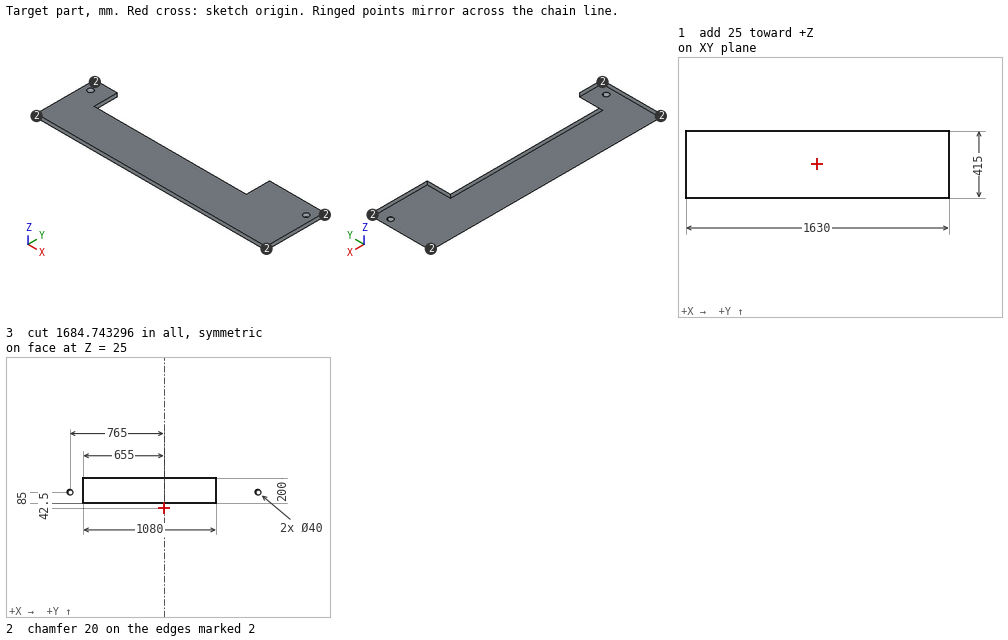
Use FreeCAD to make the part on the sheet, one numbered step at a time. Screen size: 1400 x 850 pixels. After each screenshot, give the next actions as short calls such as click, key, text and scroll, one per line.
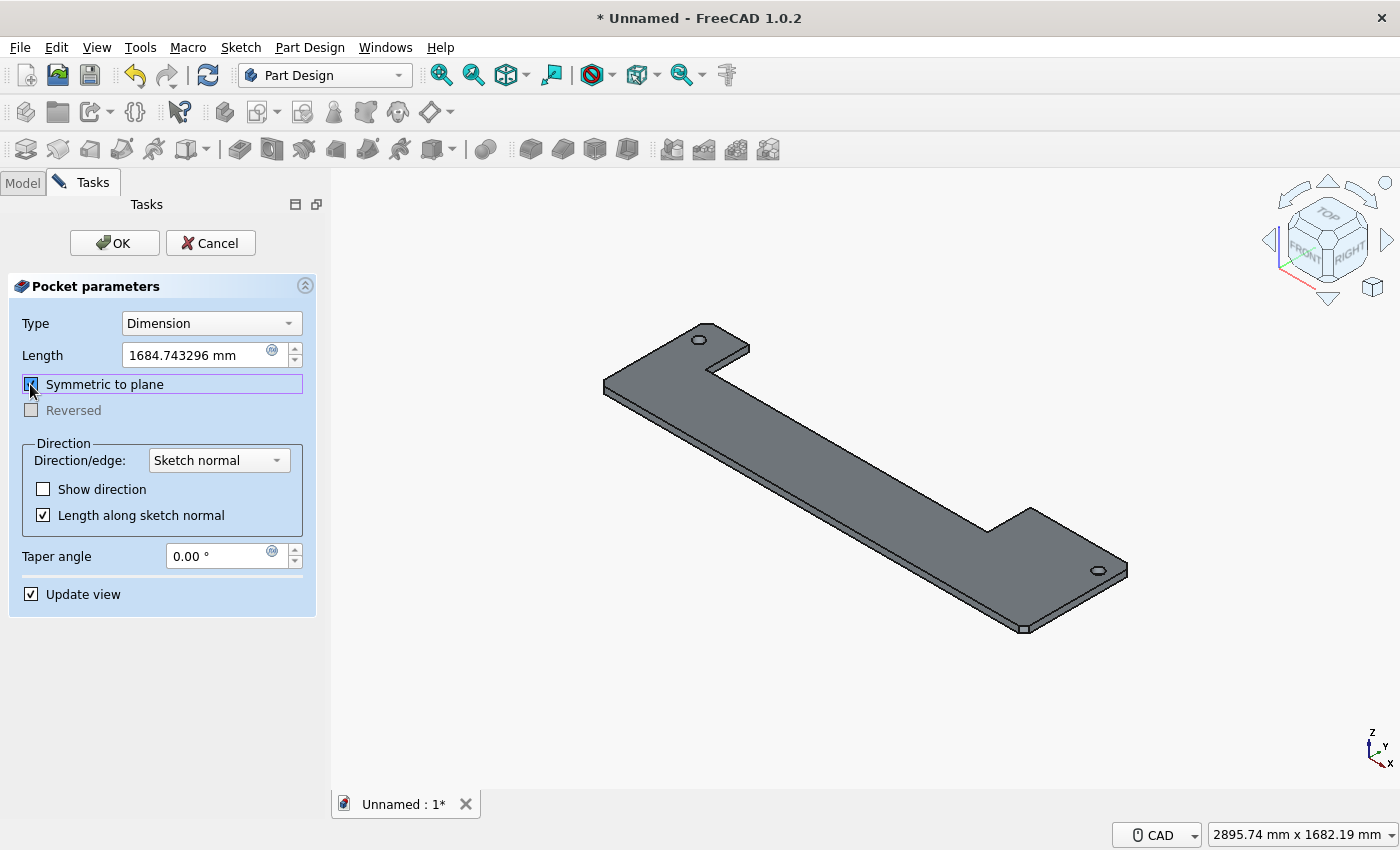
click(115, 243)